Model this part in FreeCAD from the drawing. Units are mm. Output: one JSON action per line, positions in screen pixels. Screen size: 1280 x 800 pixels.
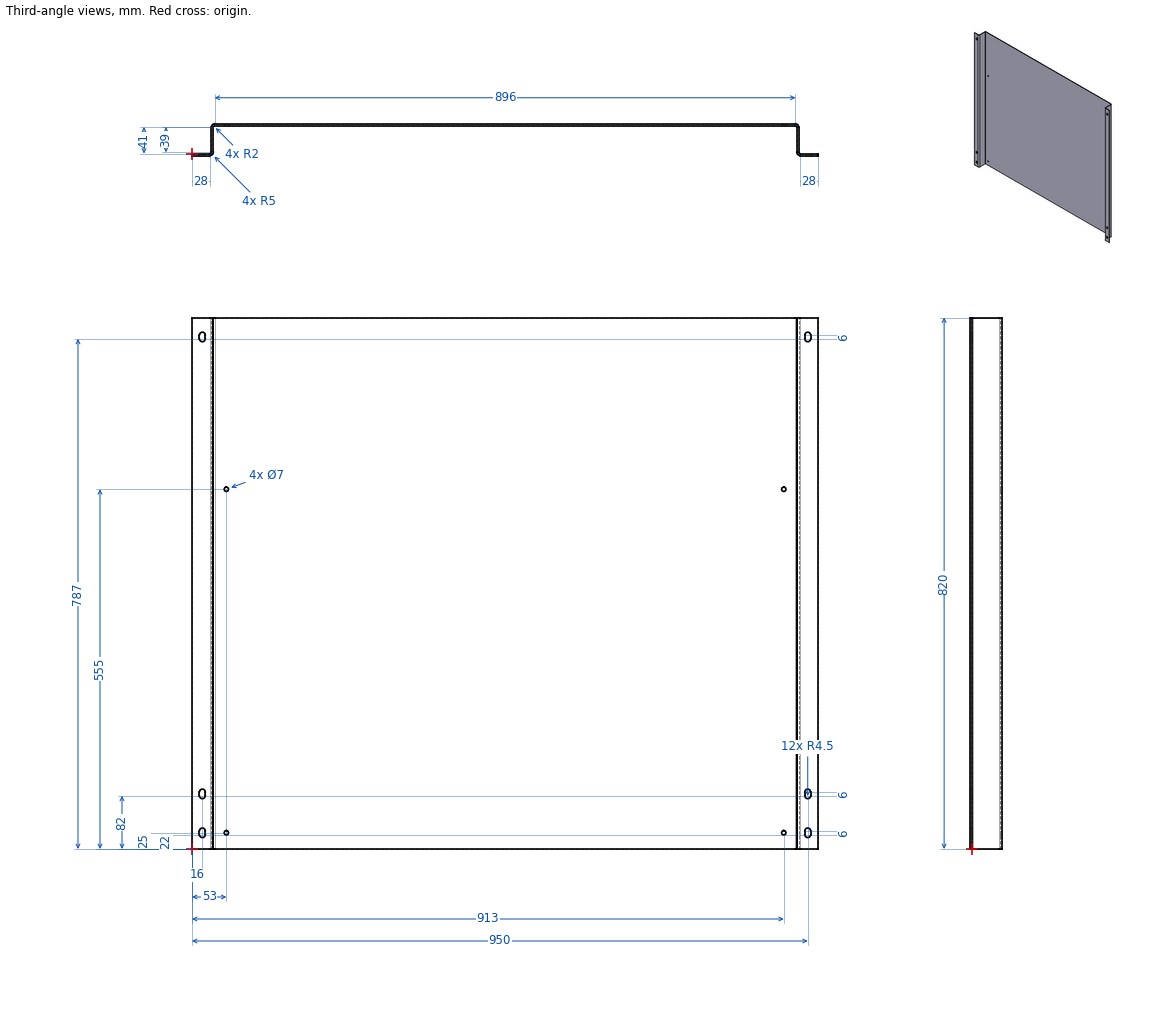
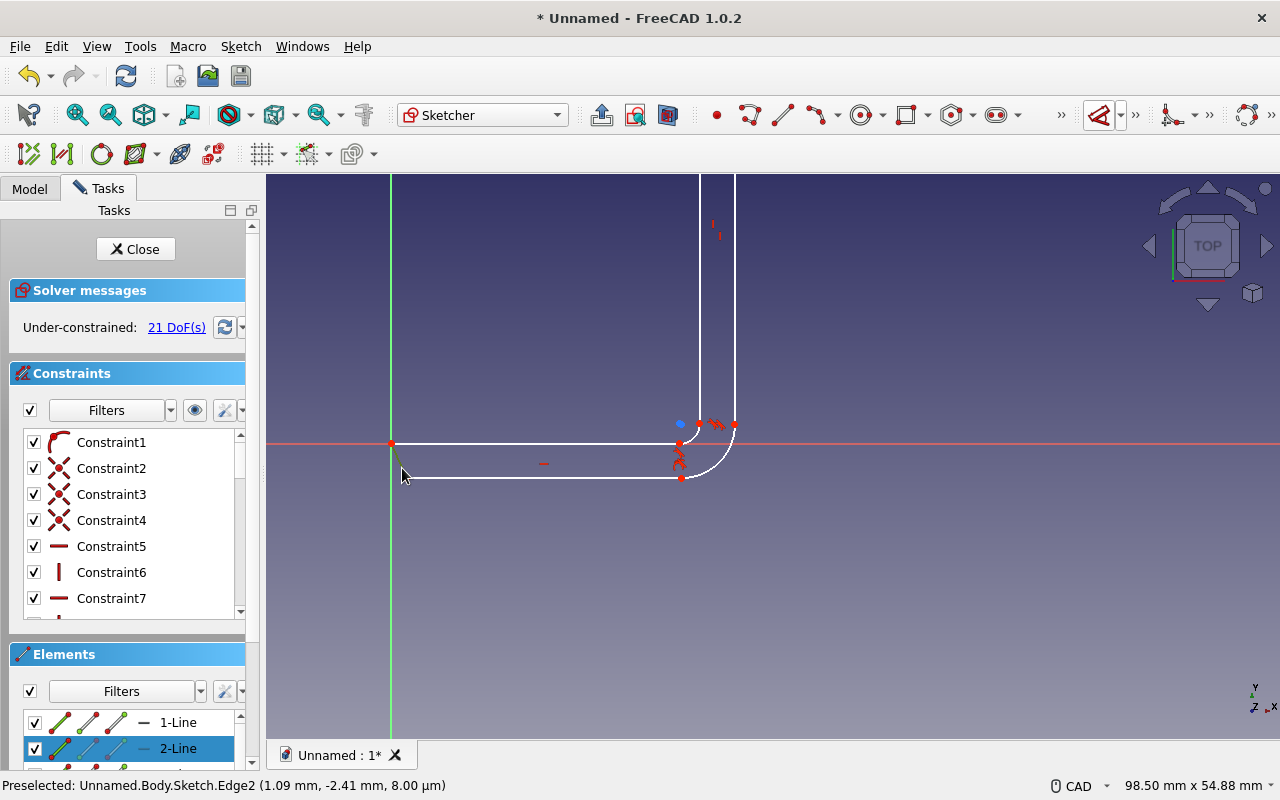
{"action": "key", "text": "v"}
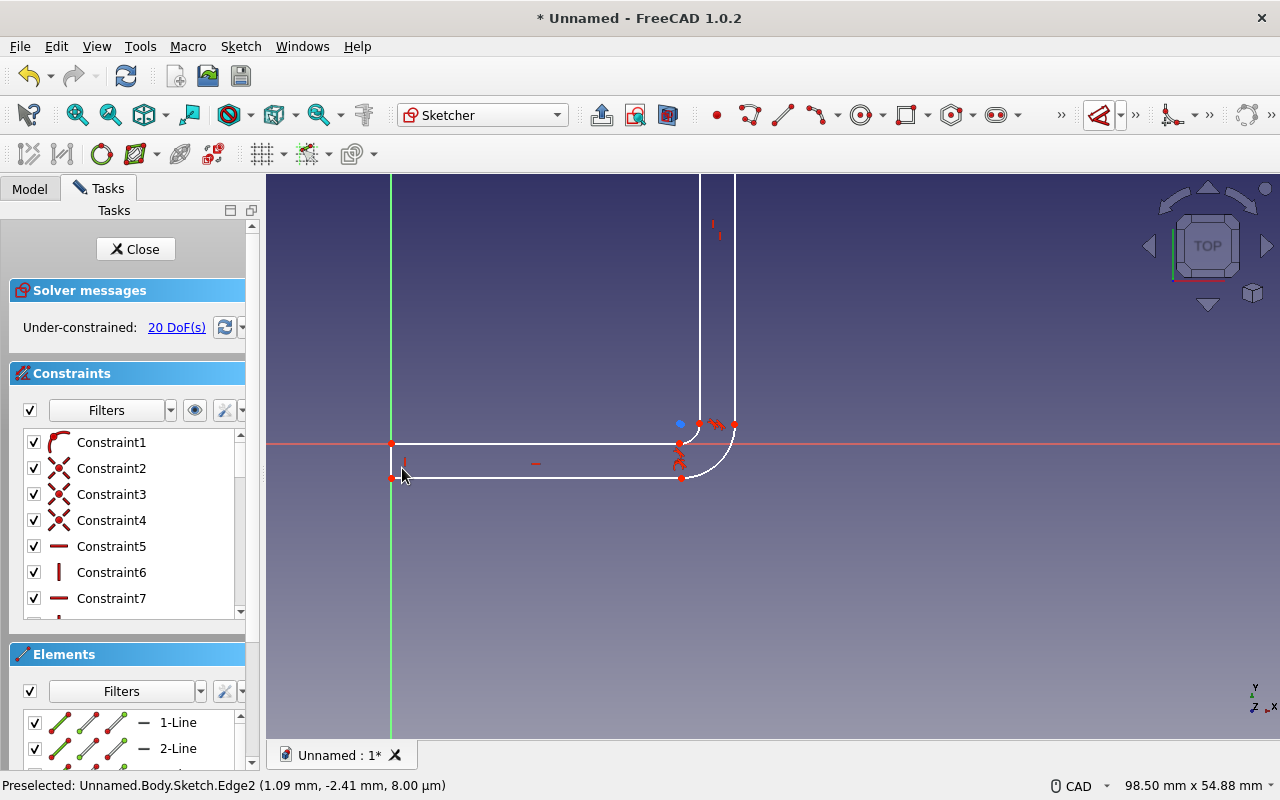
{"action": "scroll", "coordinate": [403, 472], "scroll_direction": "down", "scroll_amount": 14}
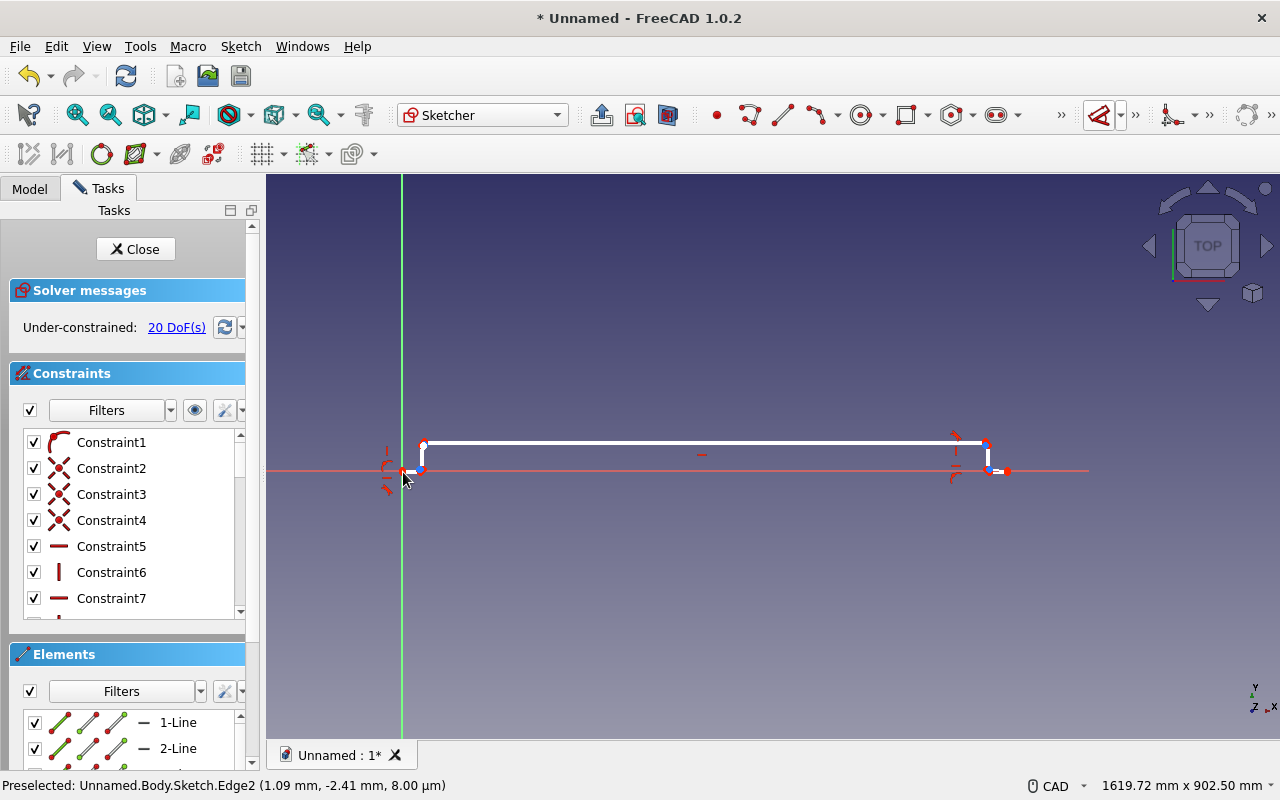
{"action": "scroll", "coordinate": [1002, 471], "scroll_direction": "up", "scroll_amount": 10}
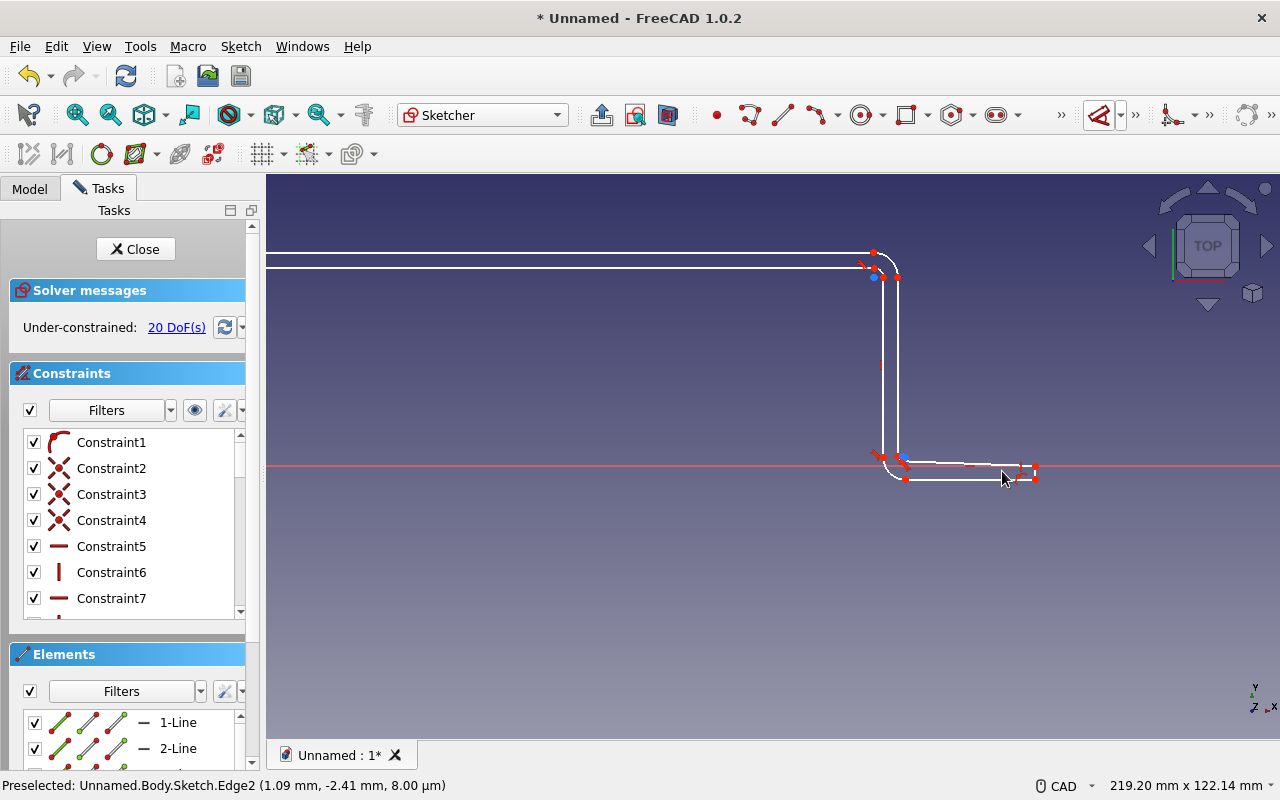
{"action": "left_click", "coordinate": [995, 465]}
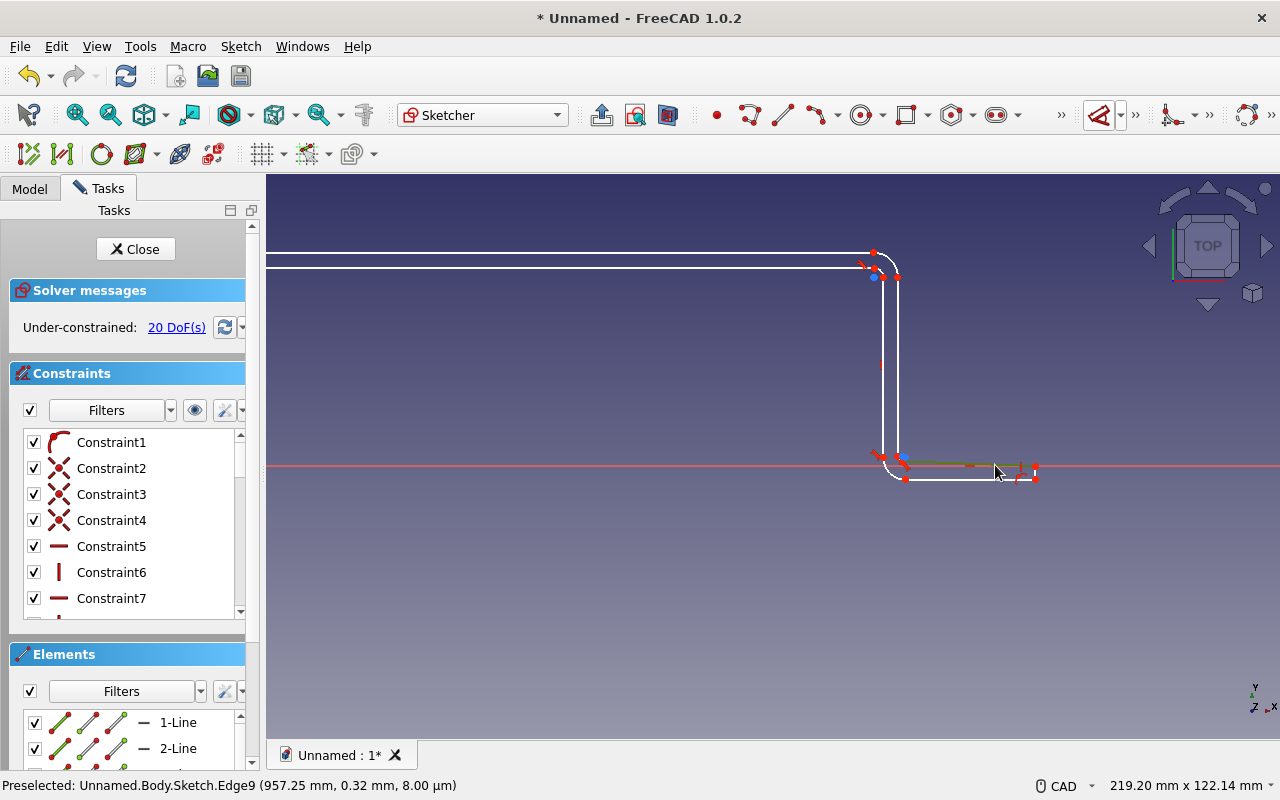
{"action": "key", "text": "h"}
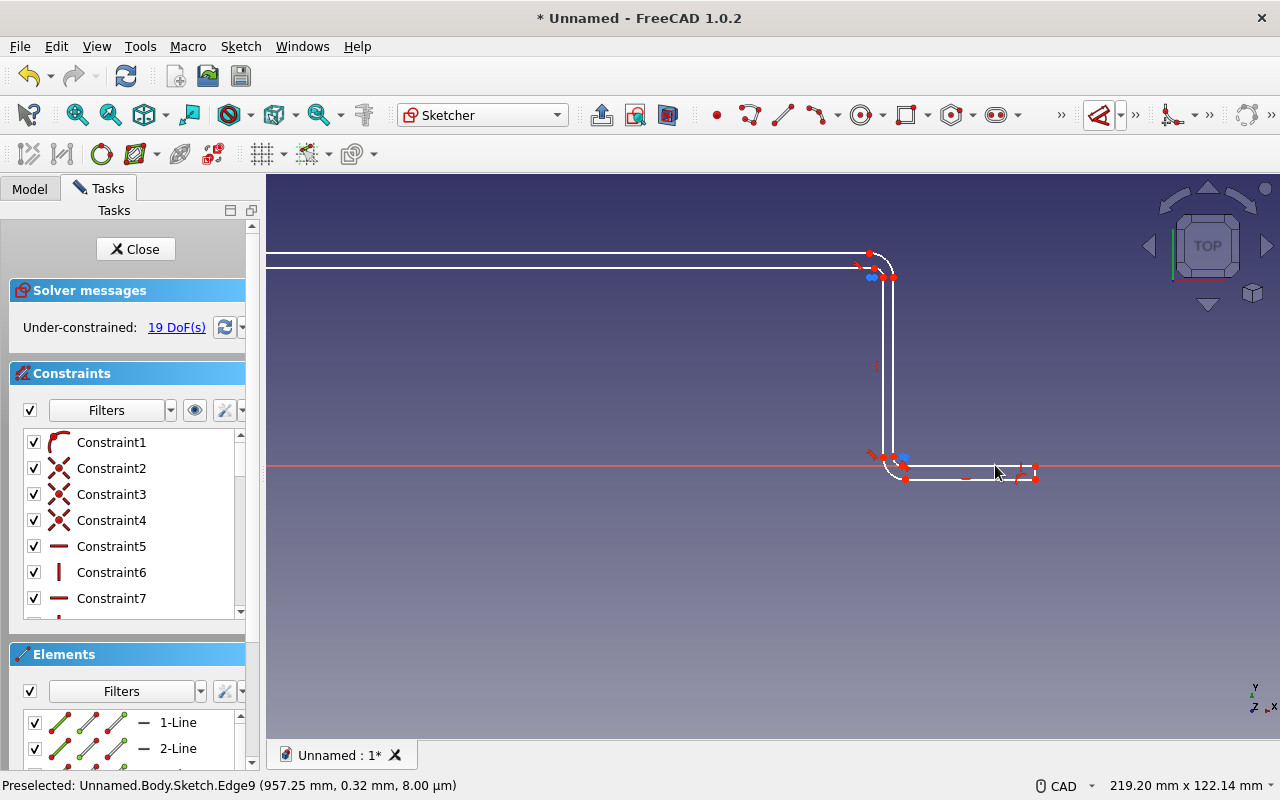
{"action": "scroll", "coordinate": [886, 468], "scroll_direction": "up", "scroll_amount": 2}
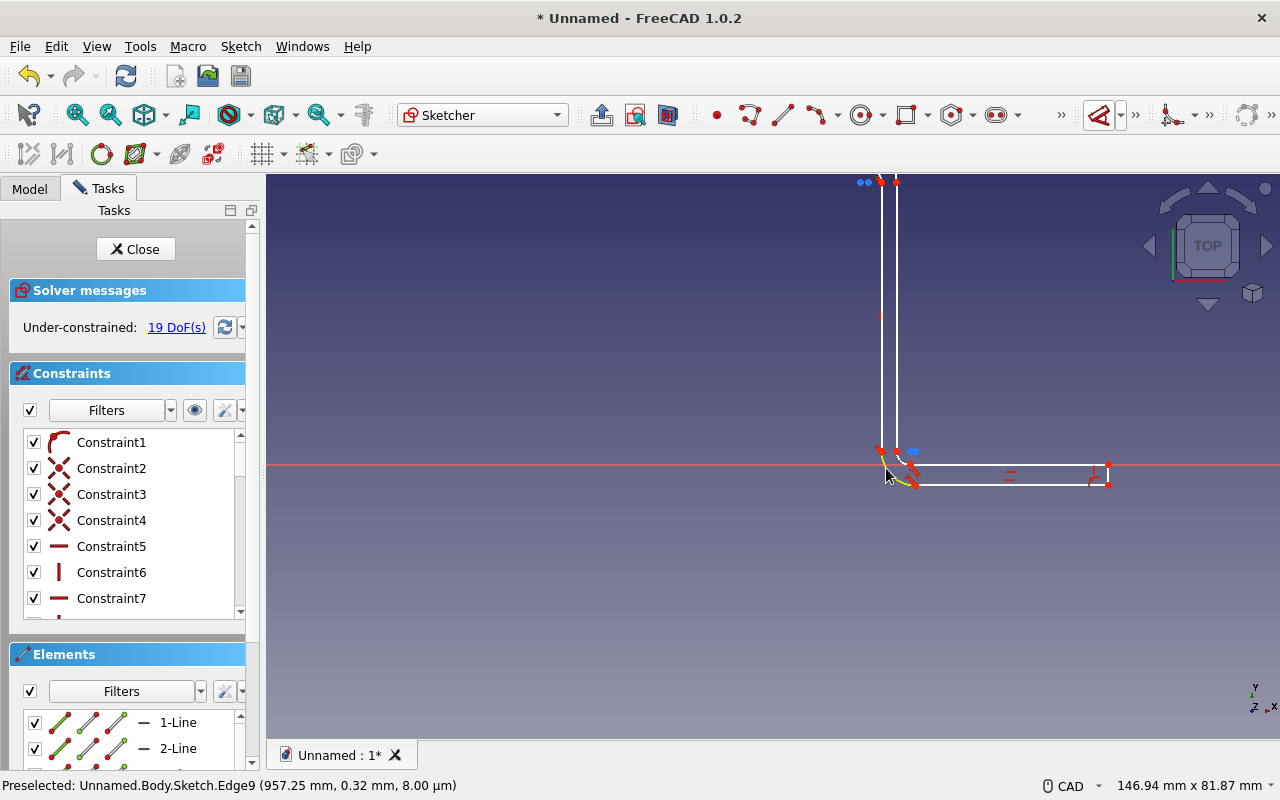
{"action": "left_click", "coordinate": [885, 467]}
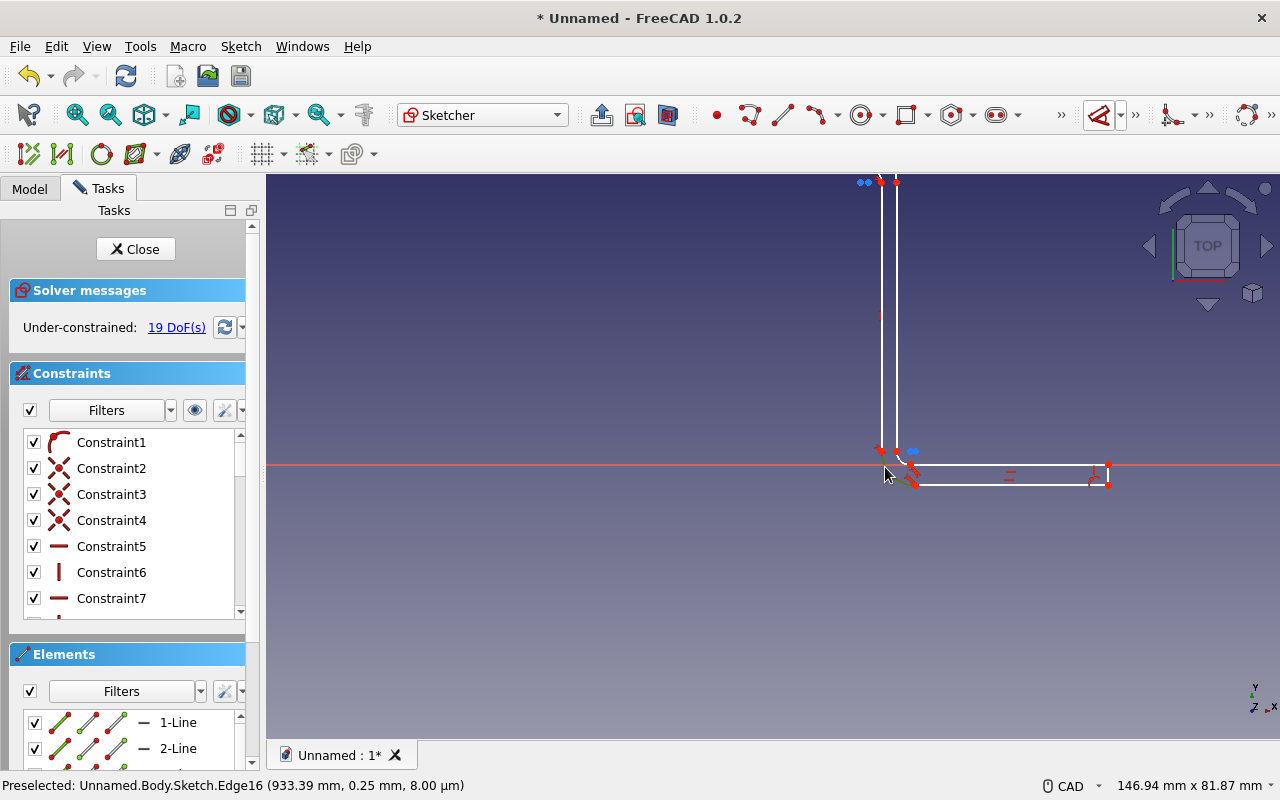
{"action": "scroll", "coordinate": [898, 457], "scroll_direction": "up", "scroll_amount": 2}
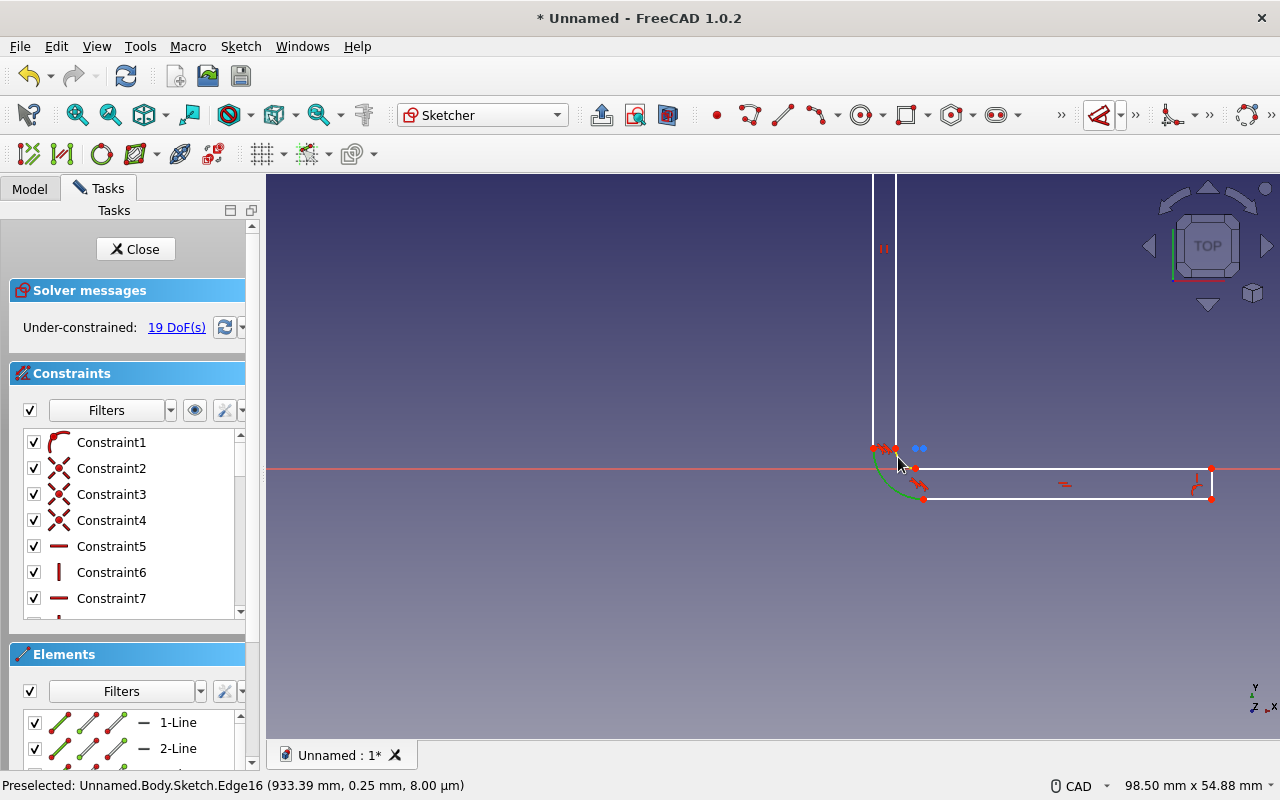
{"action": "left_click", "coordinate": [898, 457]}